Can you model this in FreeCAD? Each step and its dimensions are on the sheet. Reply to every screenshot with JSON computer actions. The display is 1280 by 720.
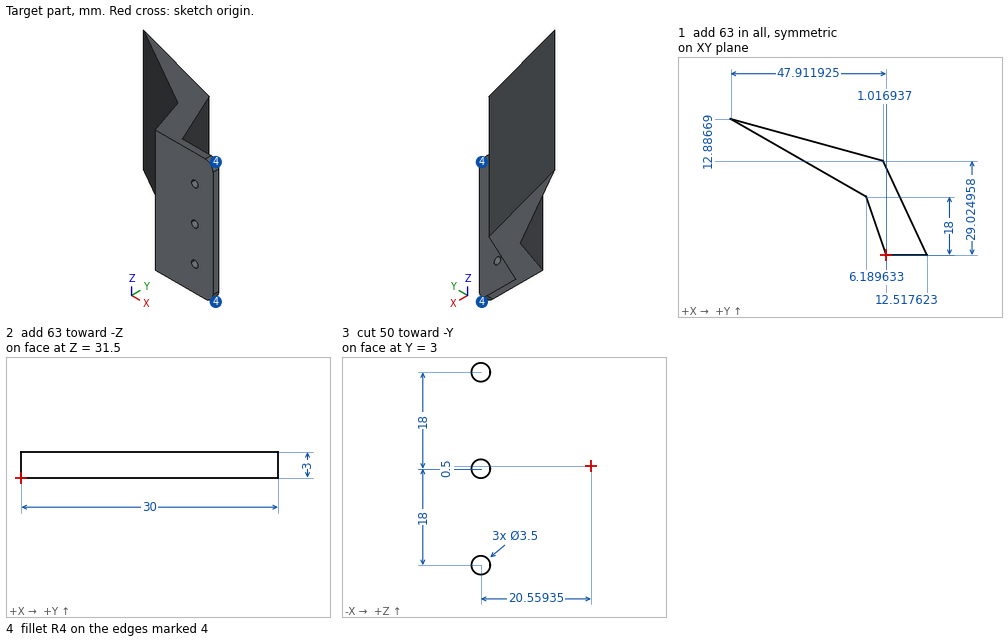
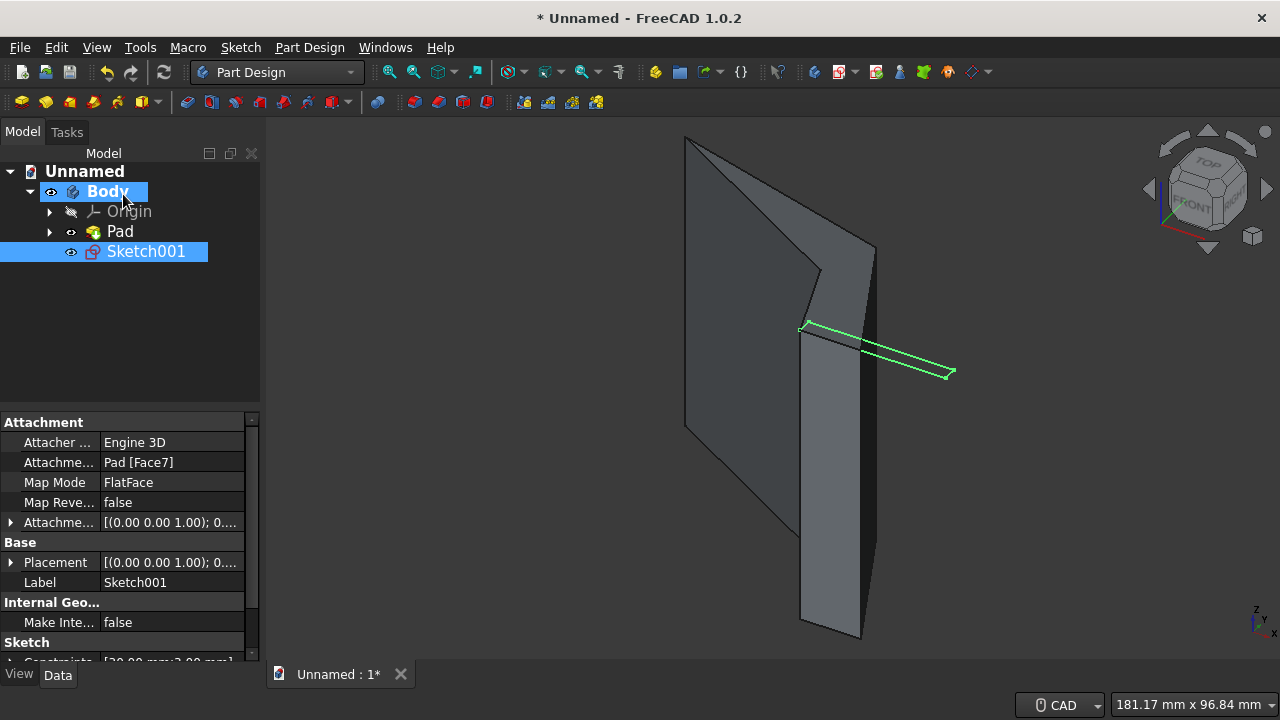
{"action": "left_click", "coordinate": [22, 102]}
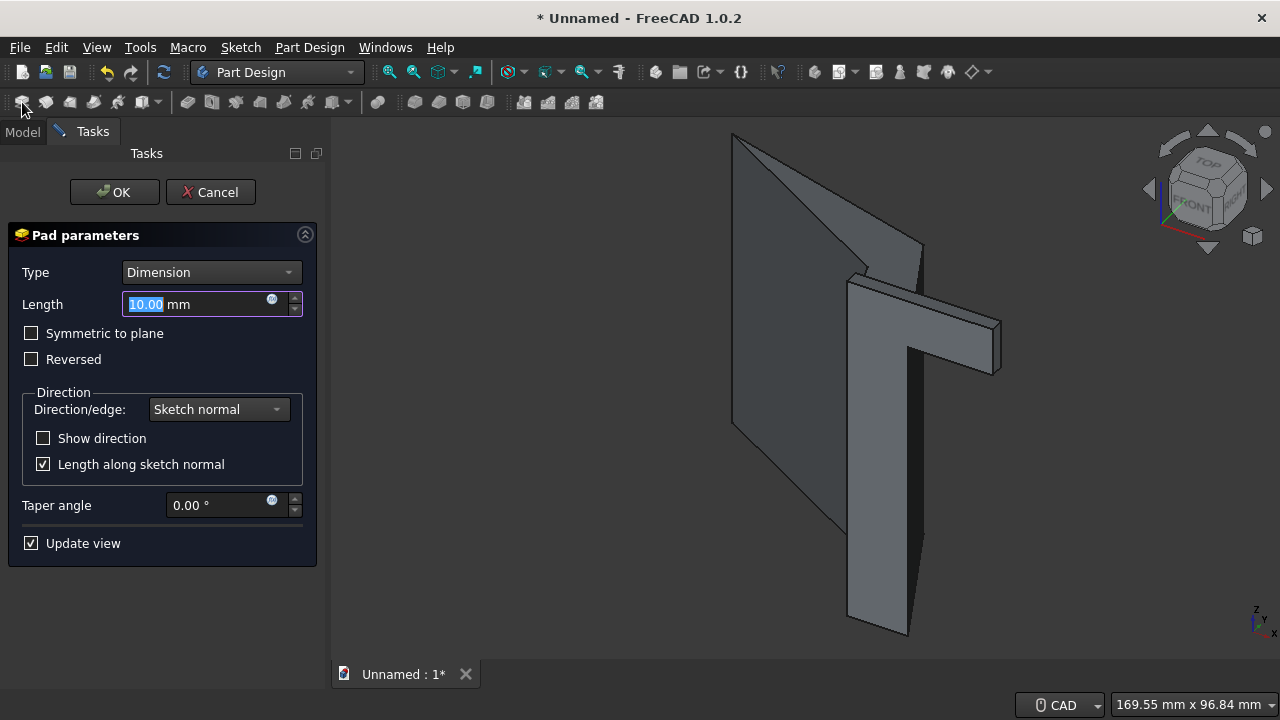
{"action": "type", "text": "63"}
{"action": "key", "text": "Tab"}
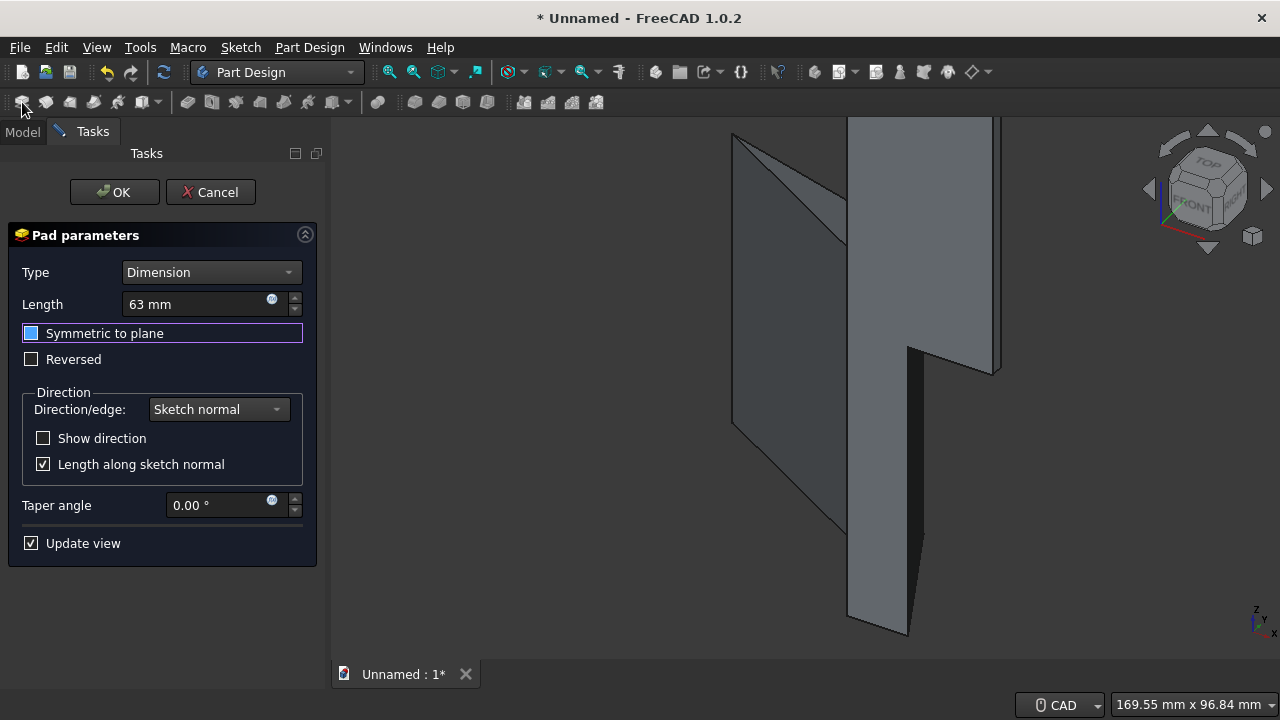
{"action": "left_click", "coordinate": [30, 359]}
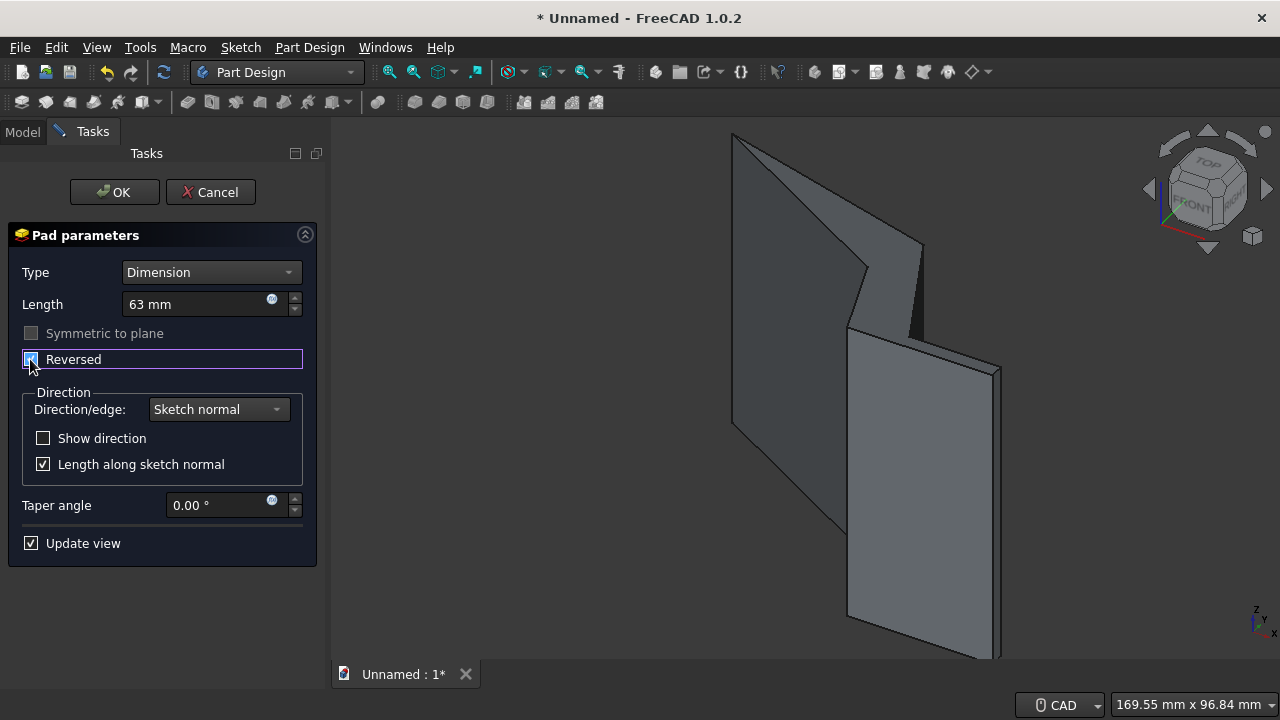
{"action": "left_click", "coordinate": [115, 192]}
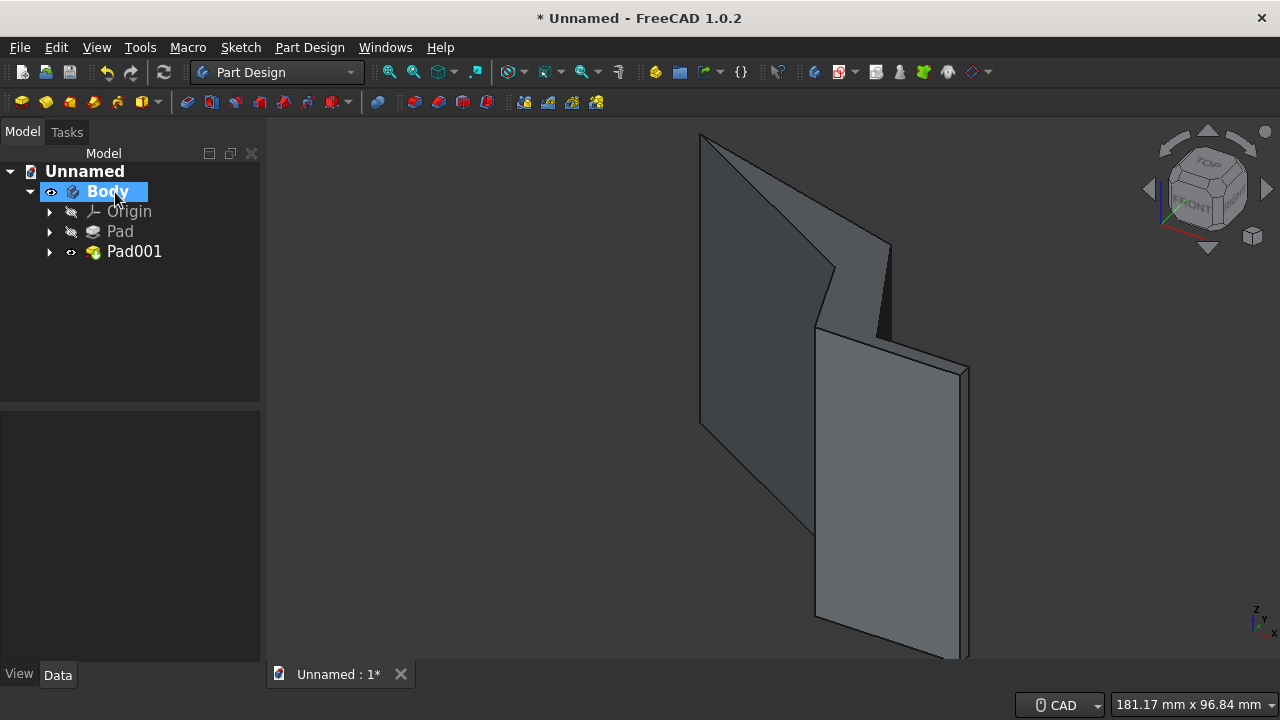
{"action": "key", "text": "v f"}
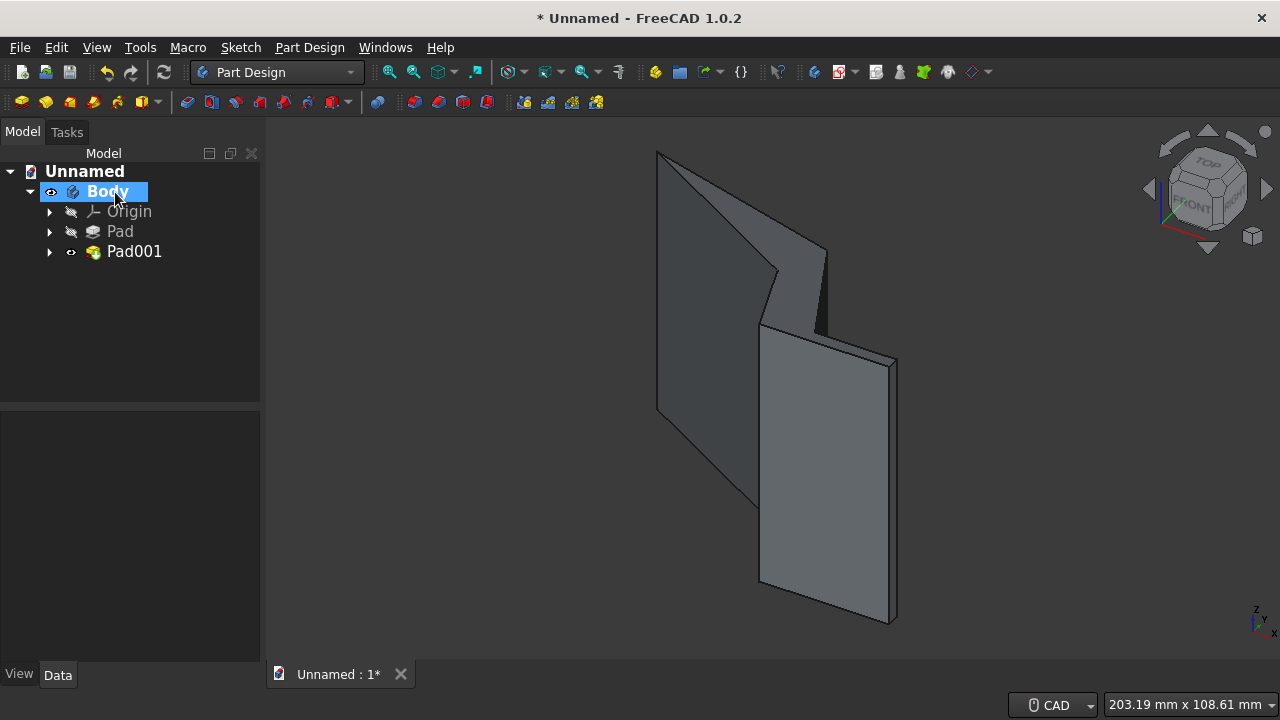
{"action": "key", "text": "4"}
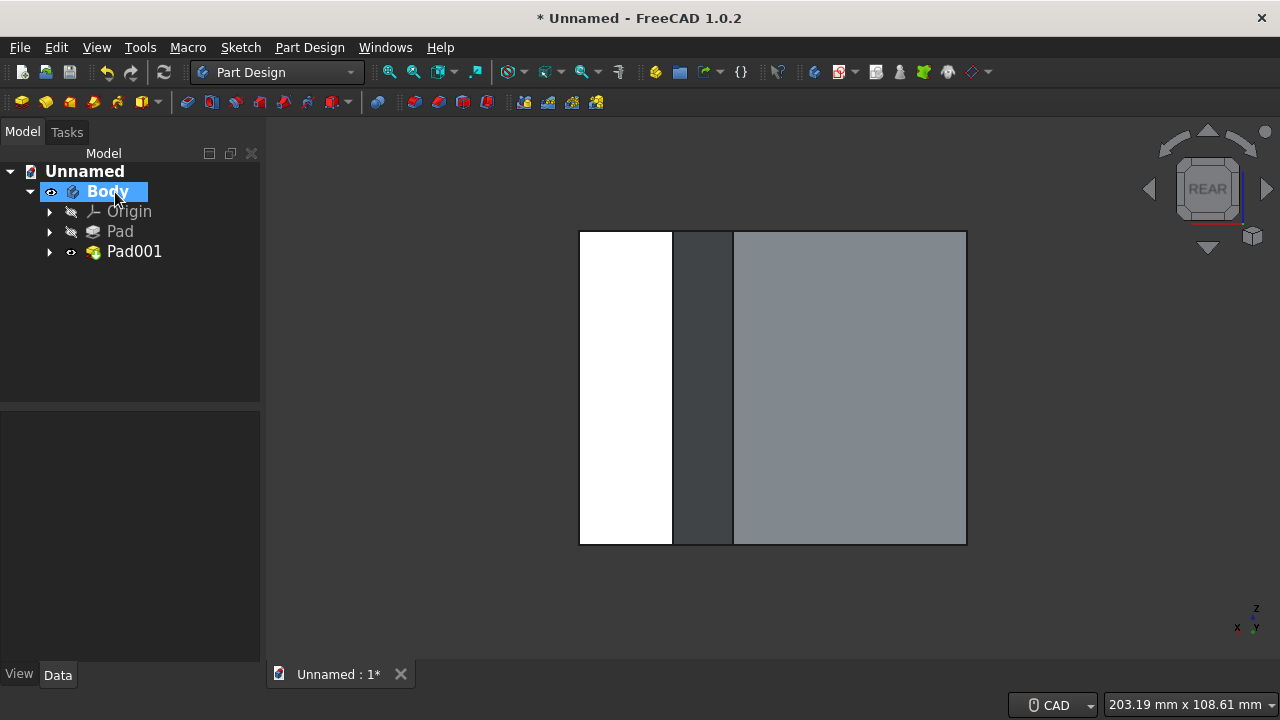
{"action": "left_click", "coordinate": [626, 297]}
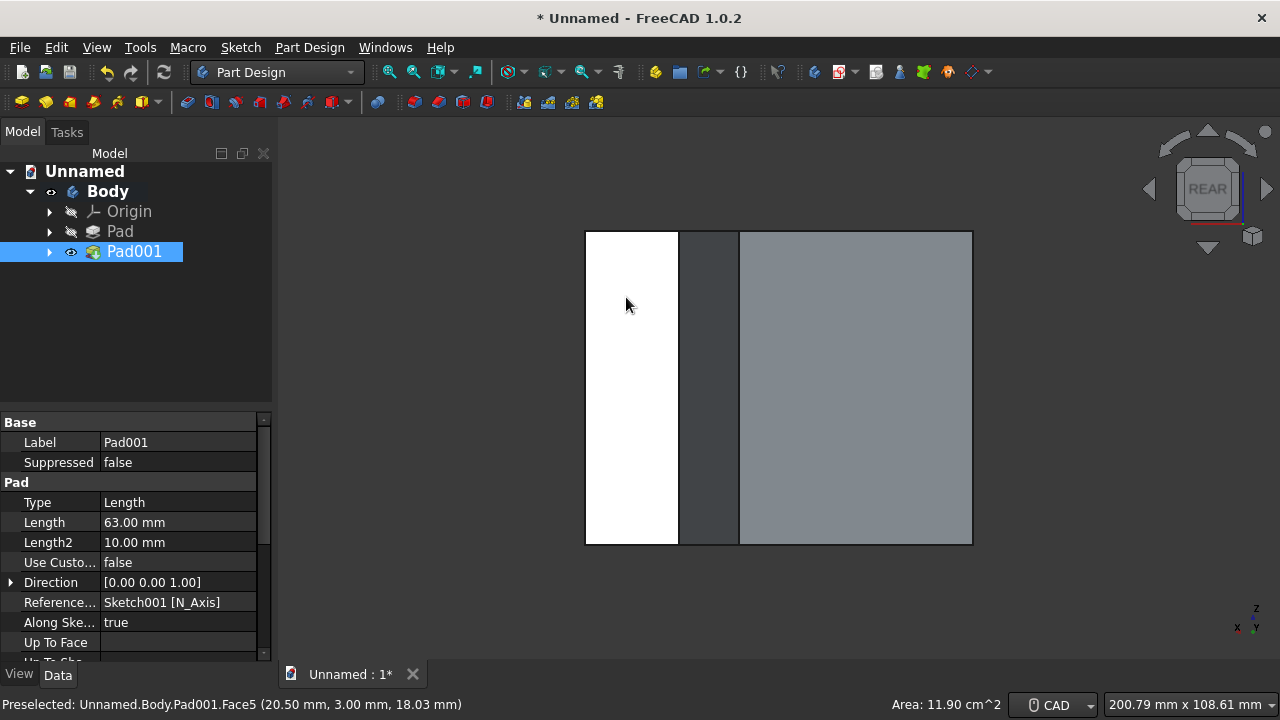
{"action": "left_click", "coordinate": [840, 72]}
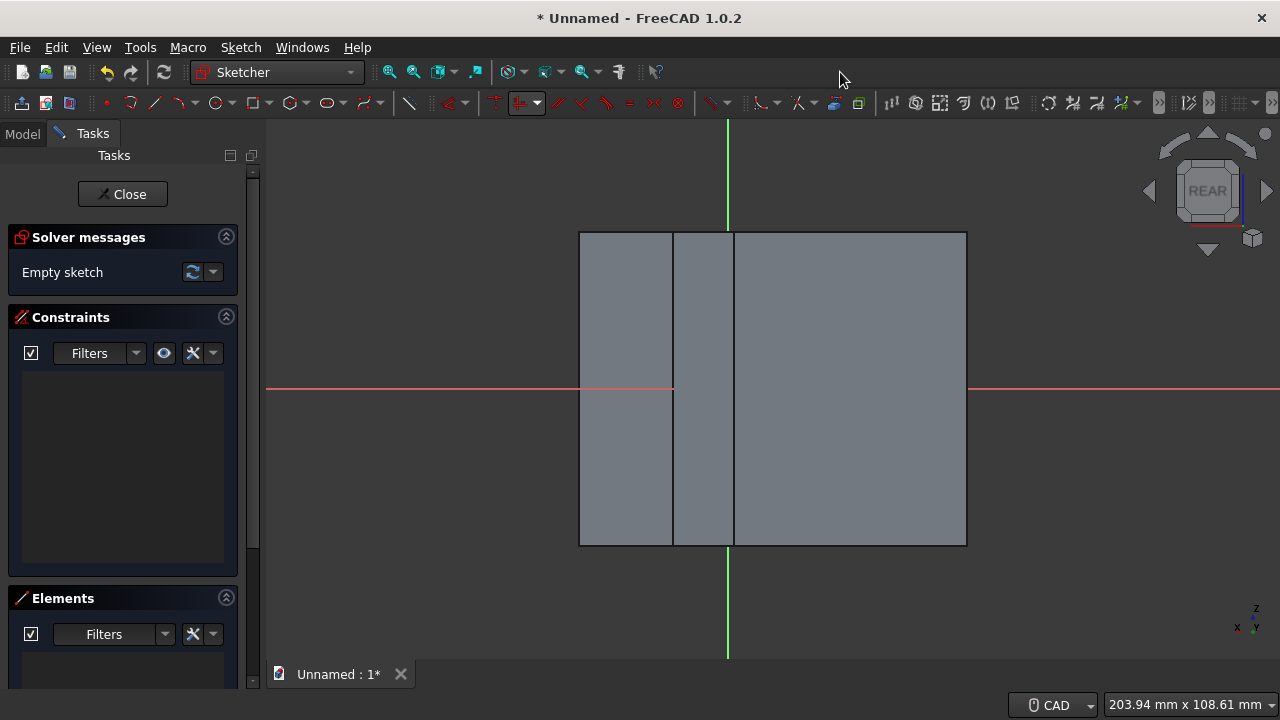
{"action": "scroll", "coordinate": [635, 395], "scroll_direction": "up", "scroll_amount": 3}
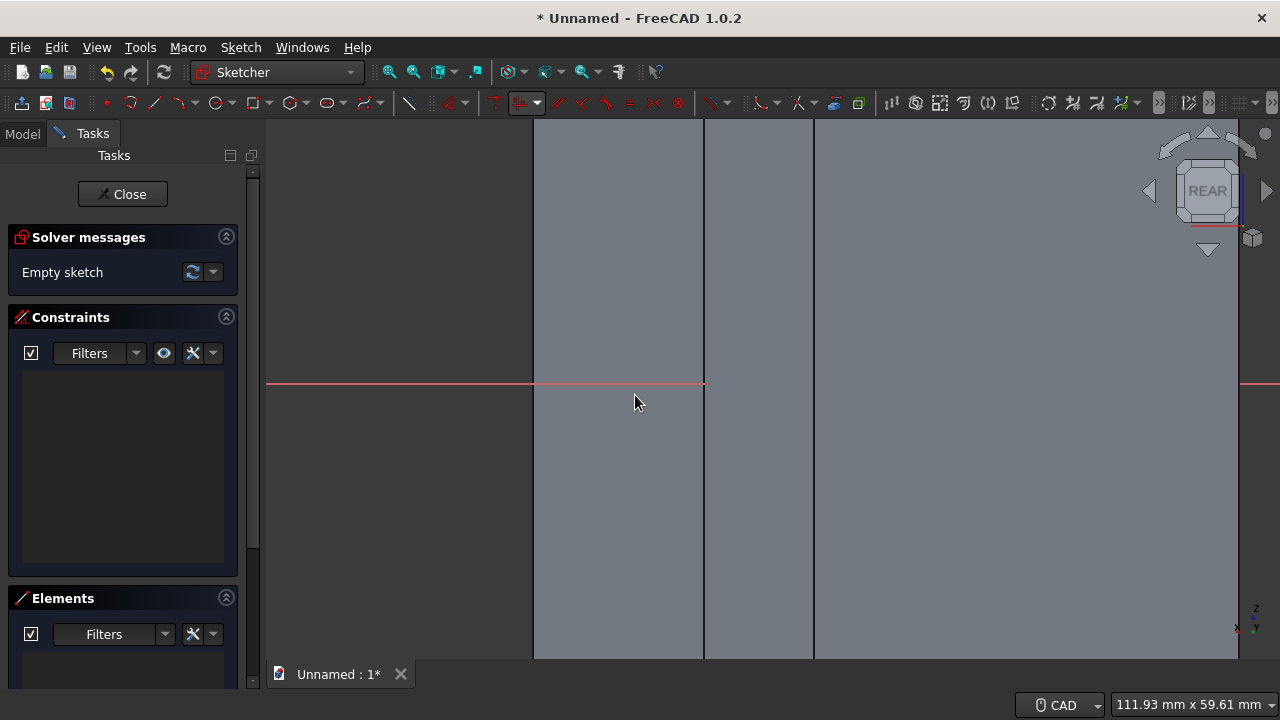
{"action": "key", "text": "g c"}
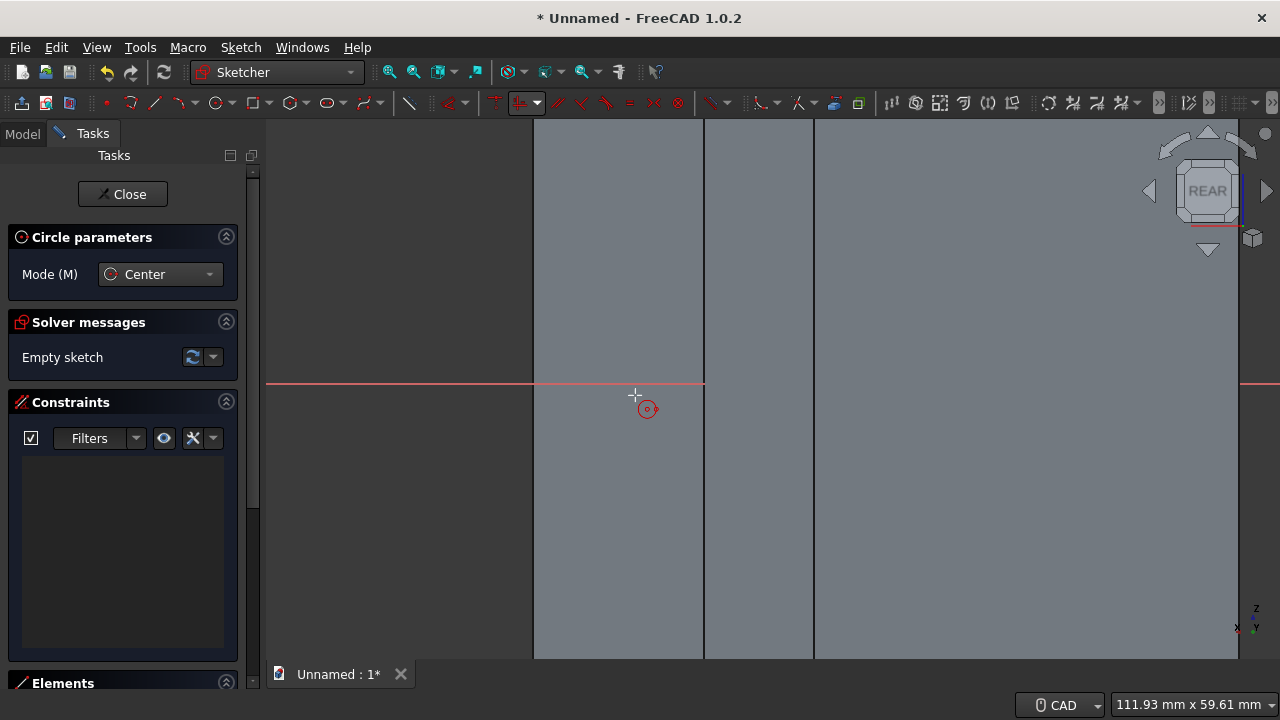
{"action": "scroll", "coordinate": [619, 551], "scroll_direction": "up", "scroll_amount": 2}